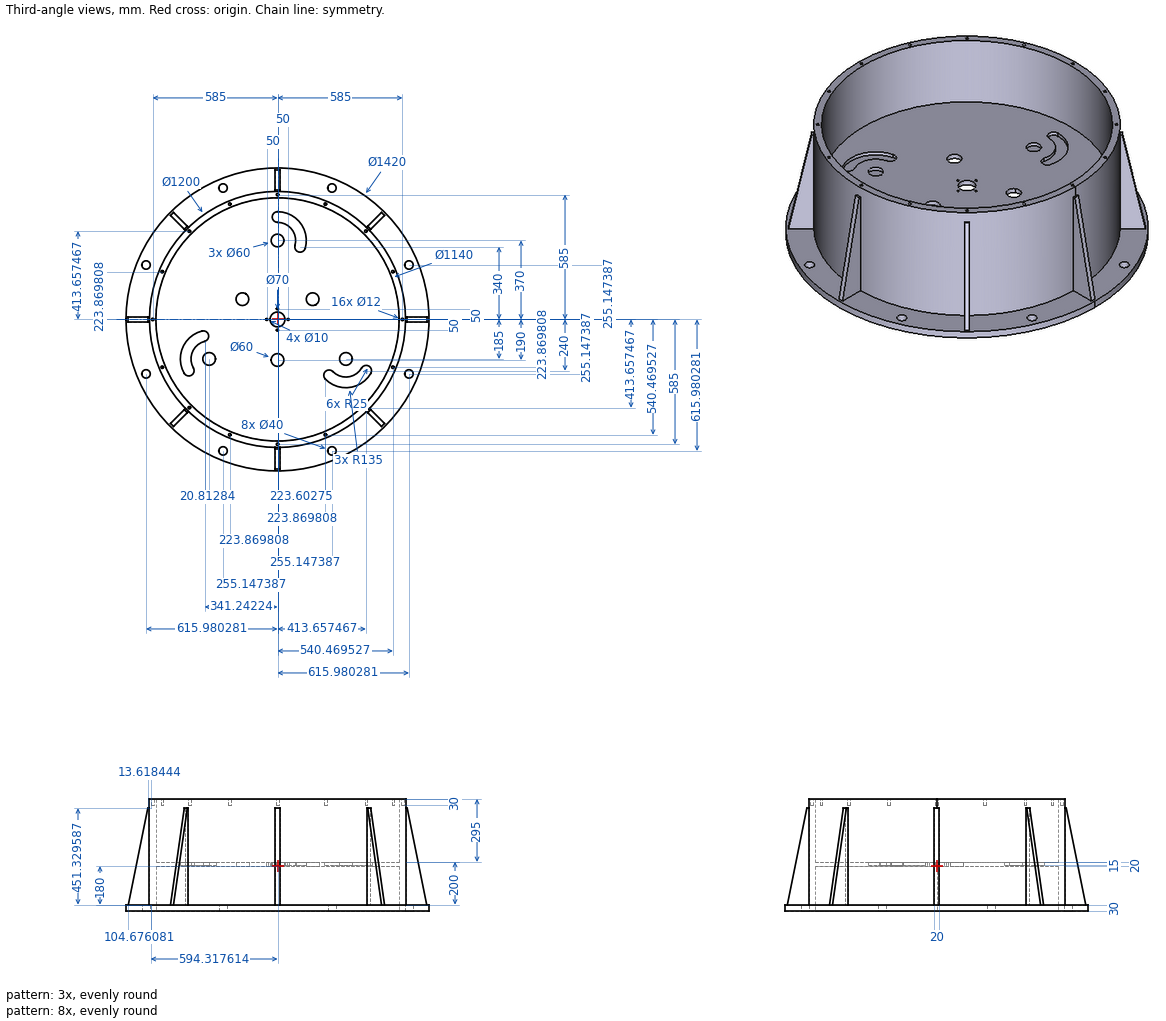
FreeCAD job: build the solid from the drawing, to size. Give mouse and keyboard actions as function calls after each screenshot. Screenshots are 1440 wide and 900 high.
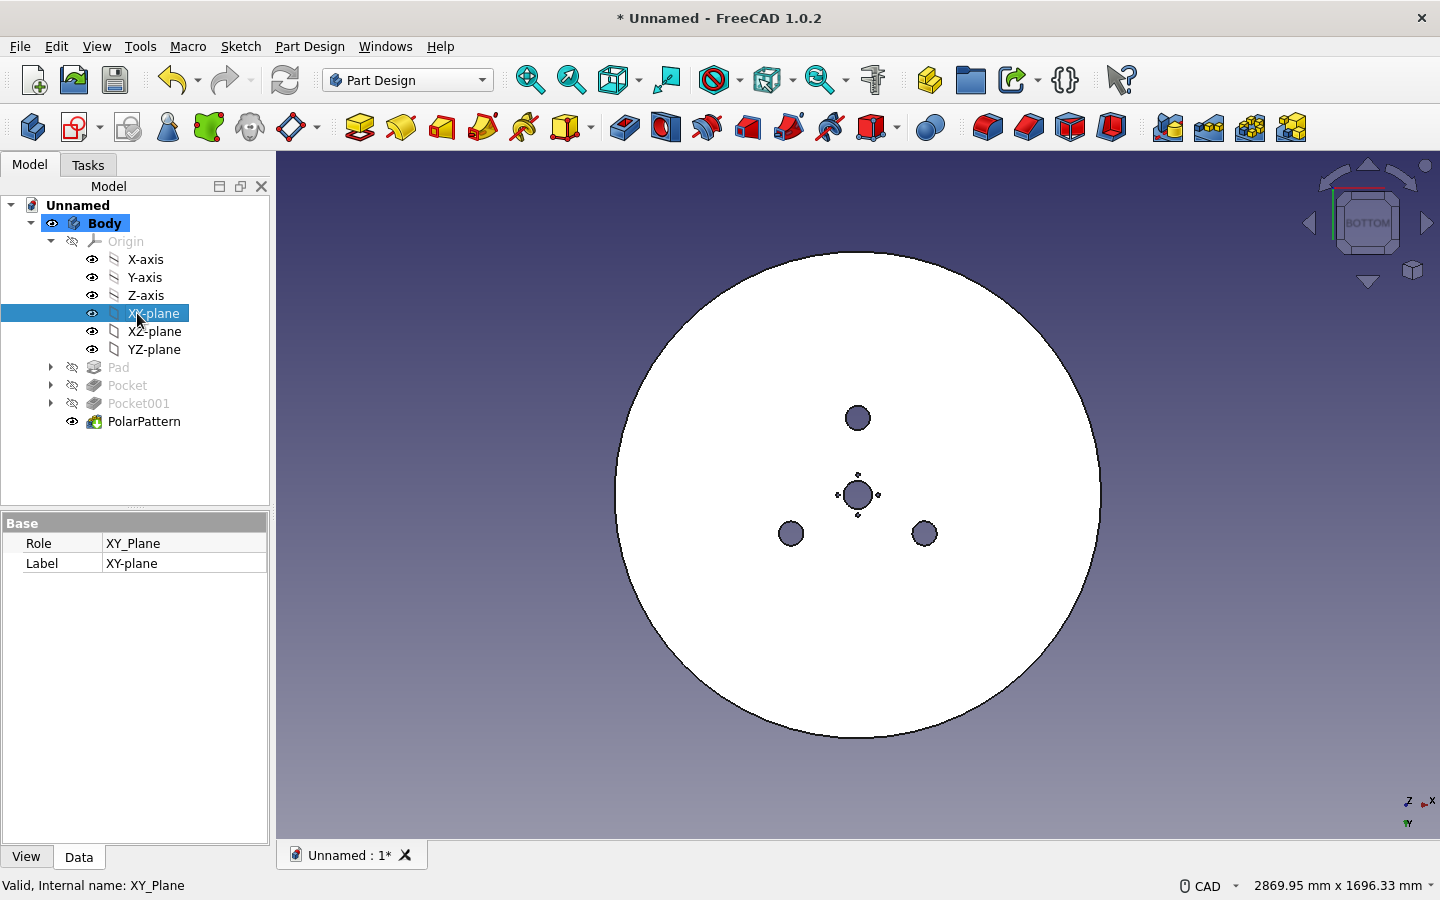
click(290, 128)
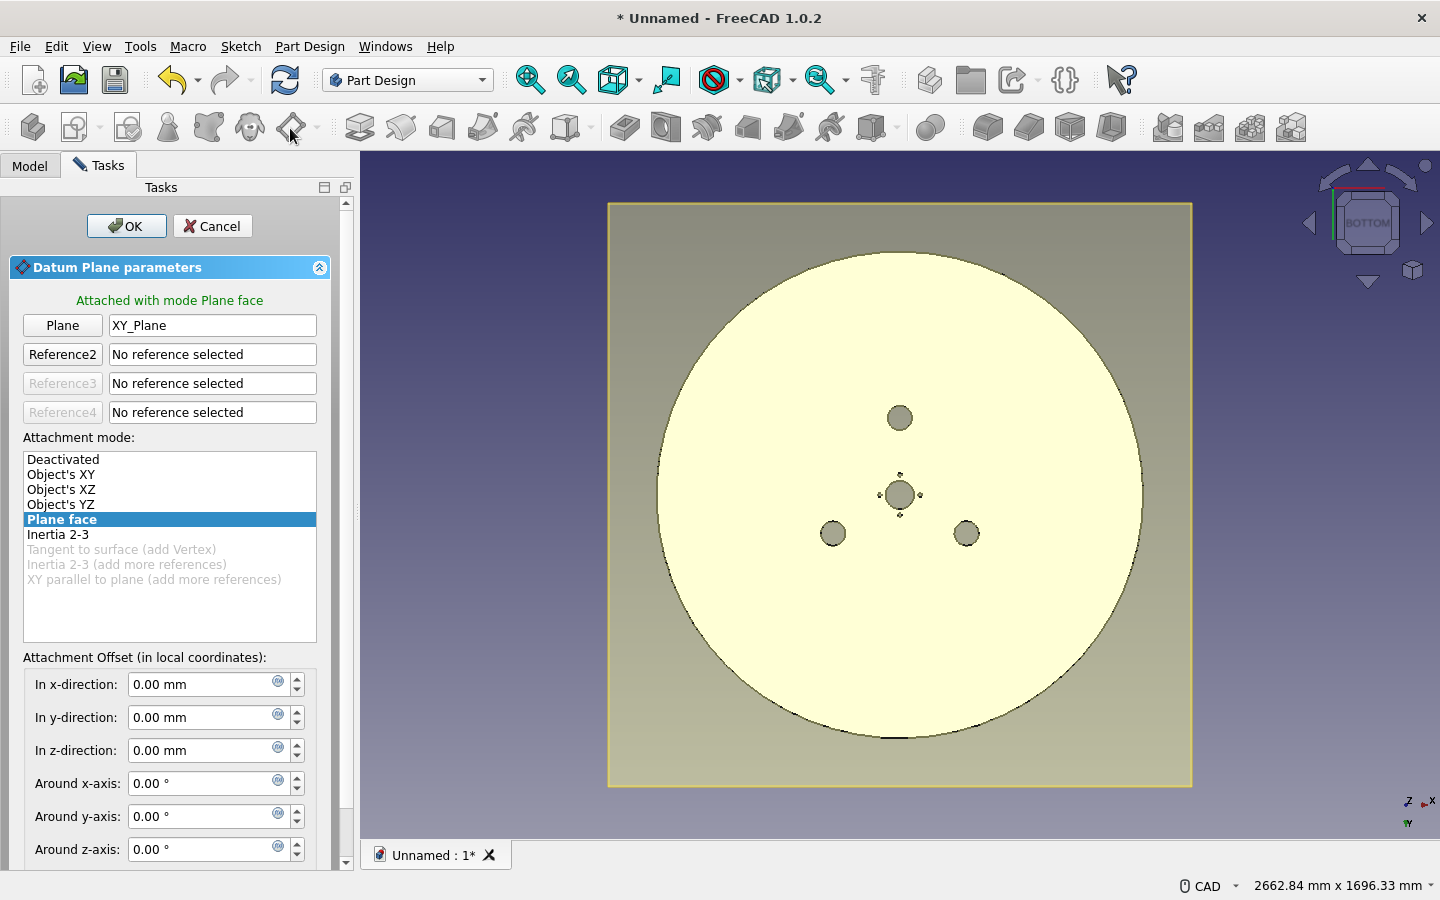
triple_click(210, 750)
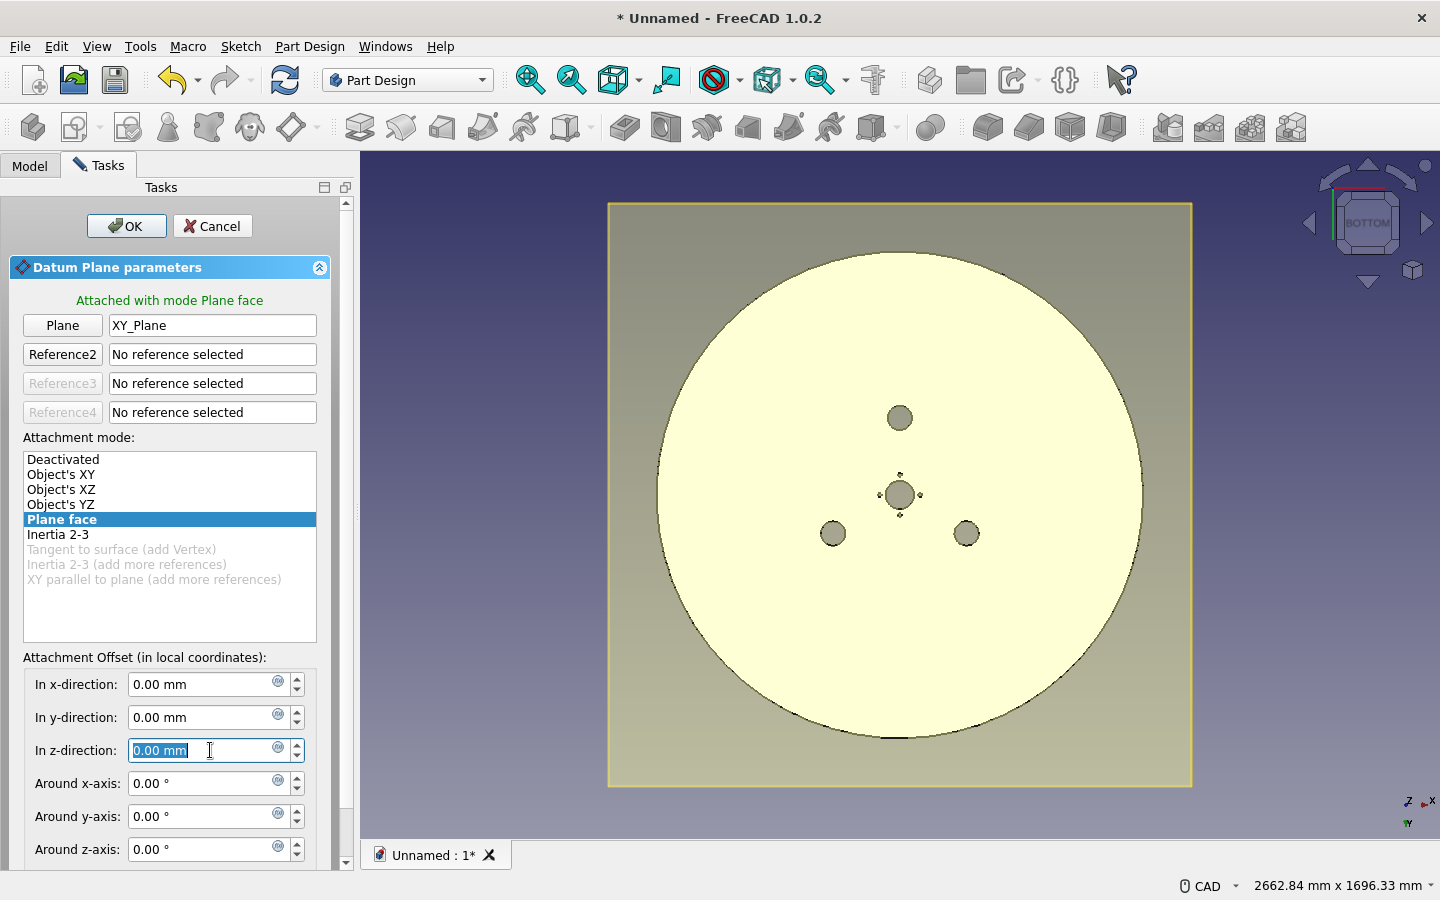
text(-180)
key(Tab)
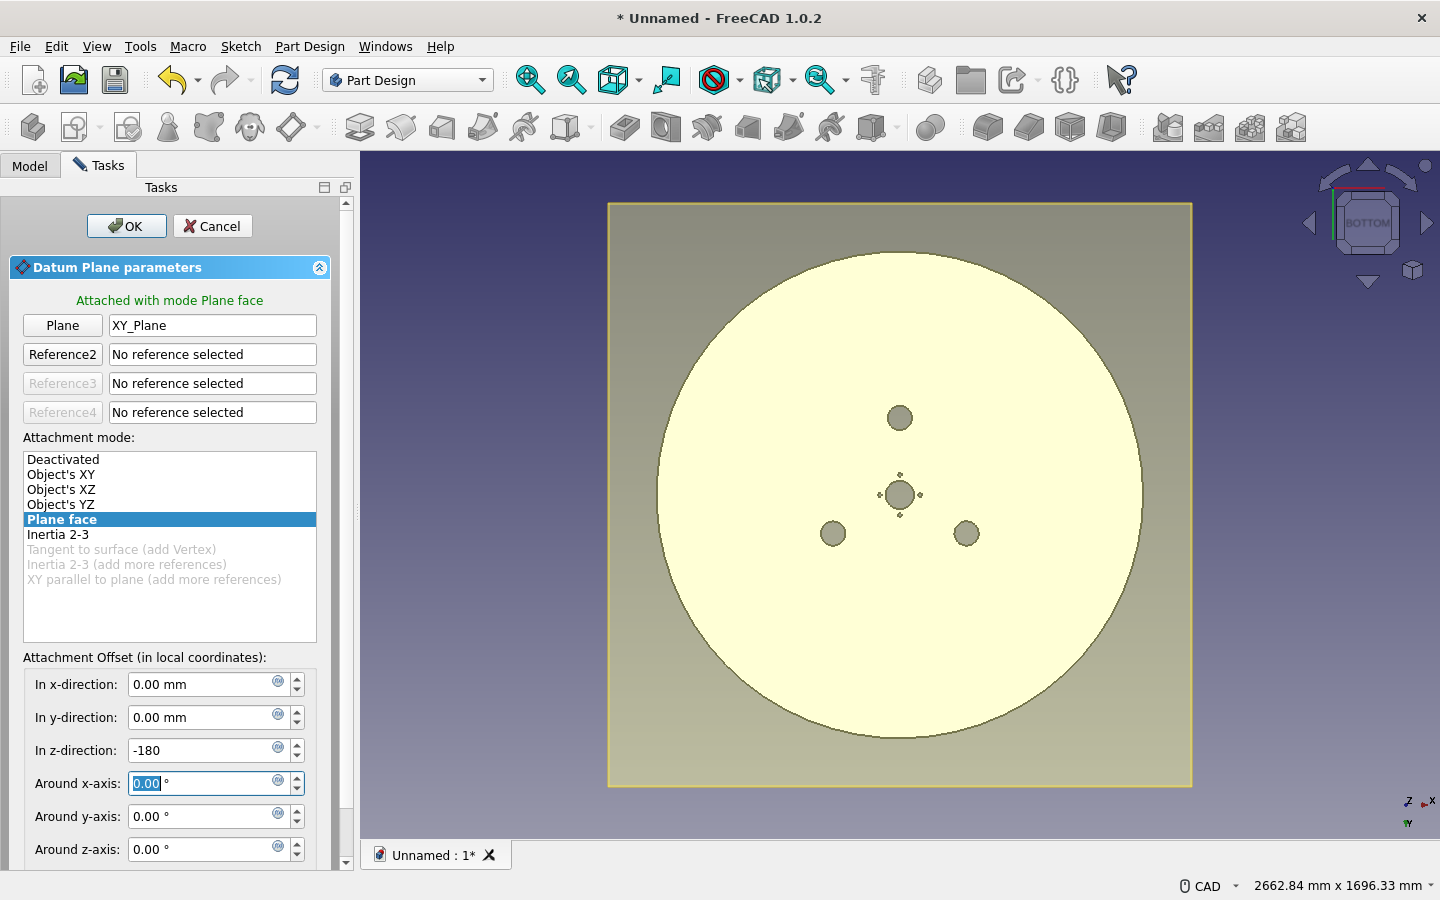
click(127, 226)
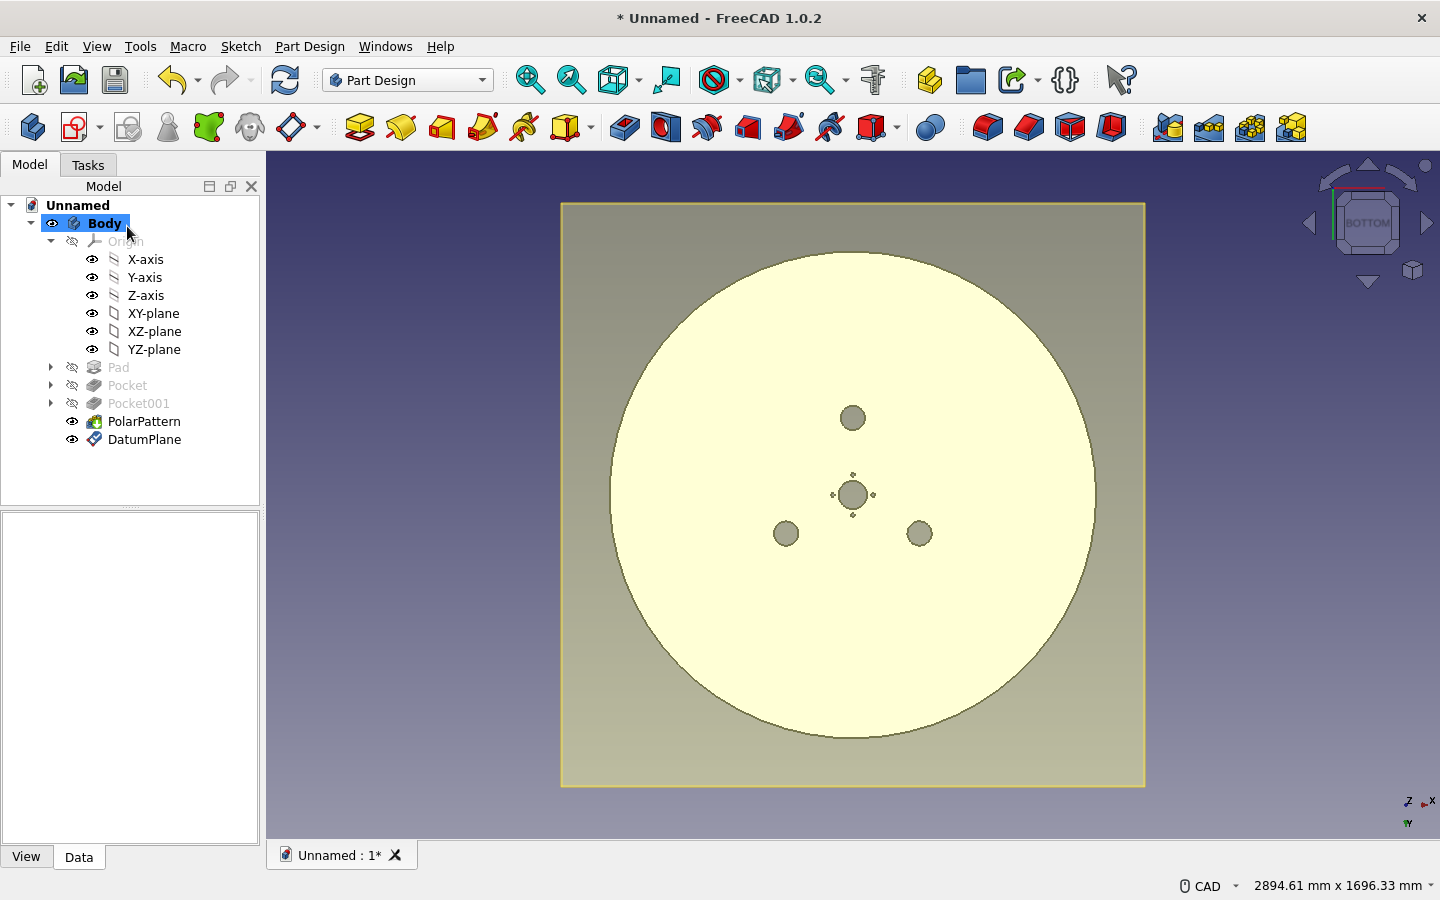
click(117, 439)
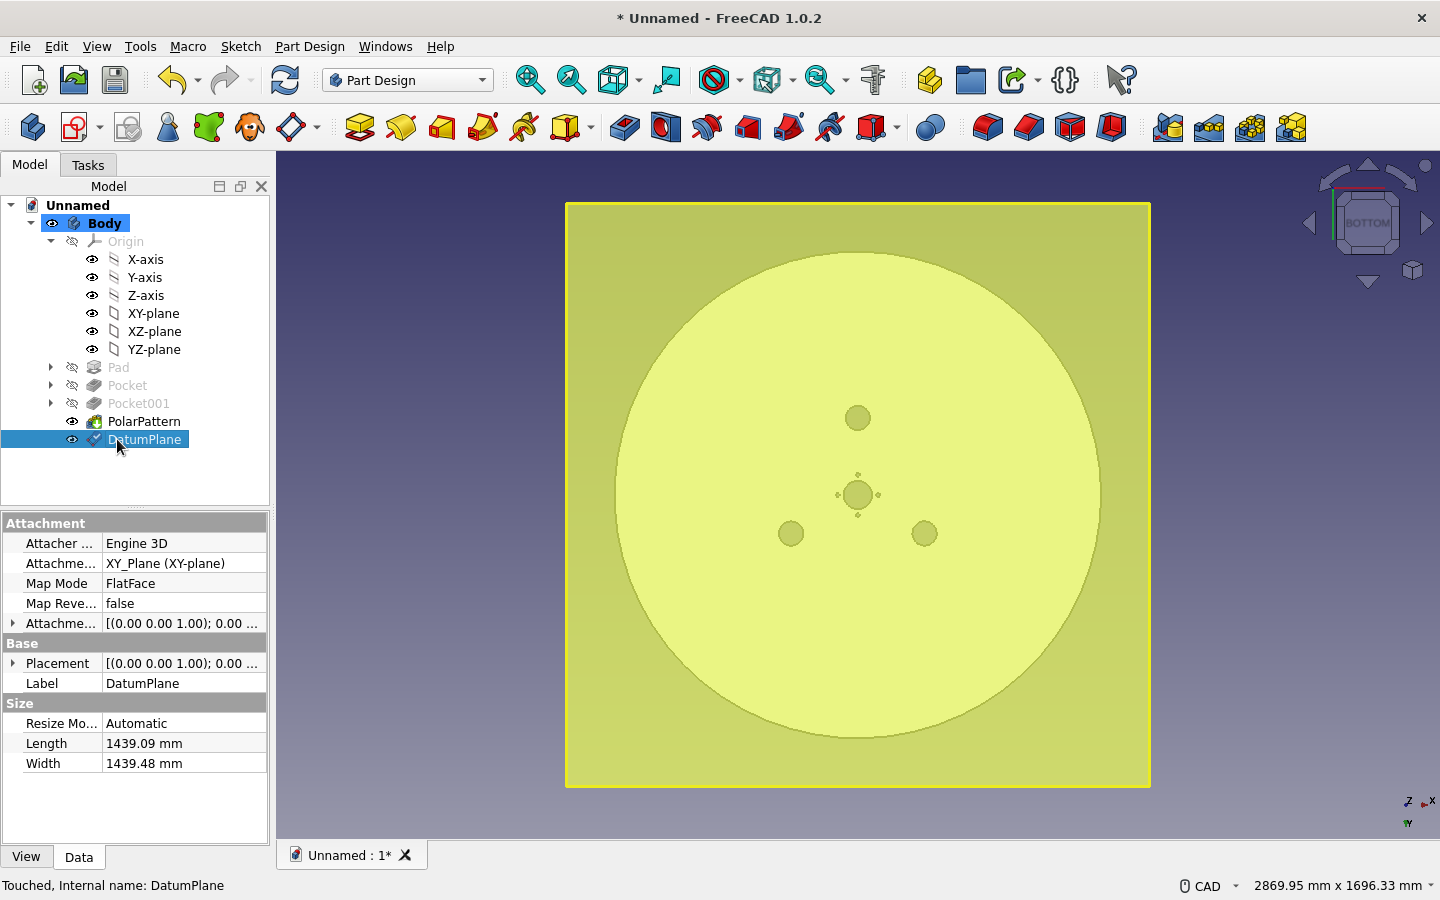
click(74, 128)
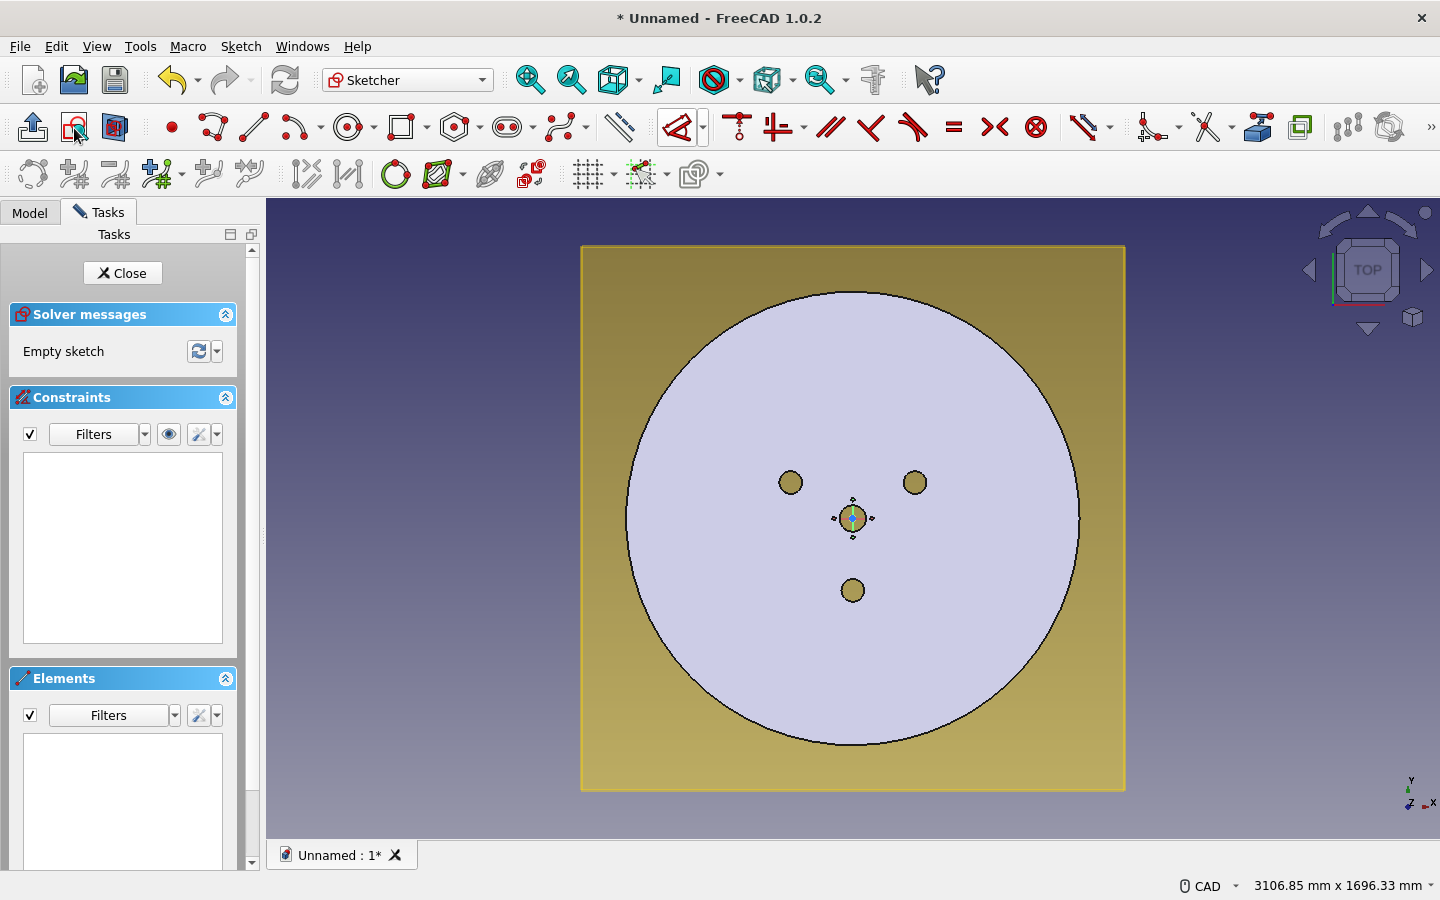
key(q)
key(s)